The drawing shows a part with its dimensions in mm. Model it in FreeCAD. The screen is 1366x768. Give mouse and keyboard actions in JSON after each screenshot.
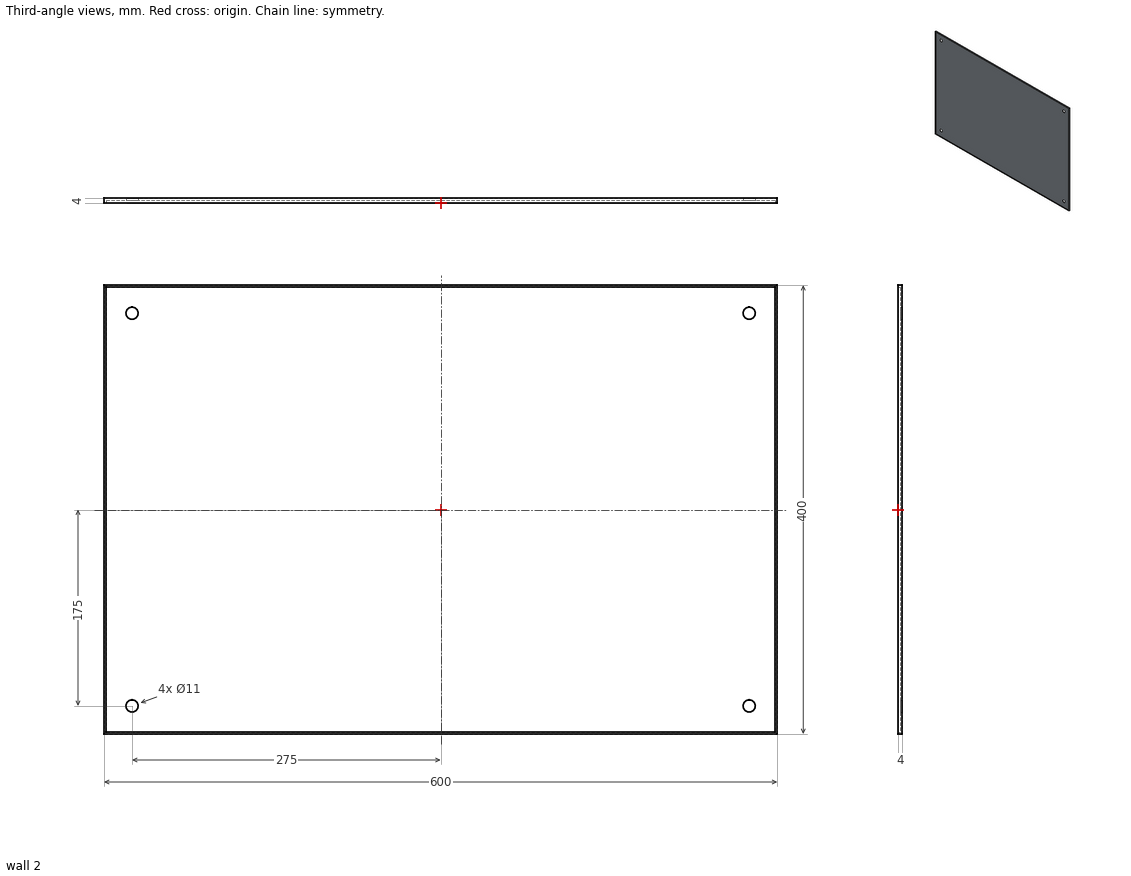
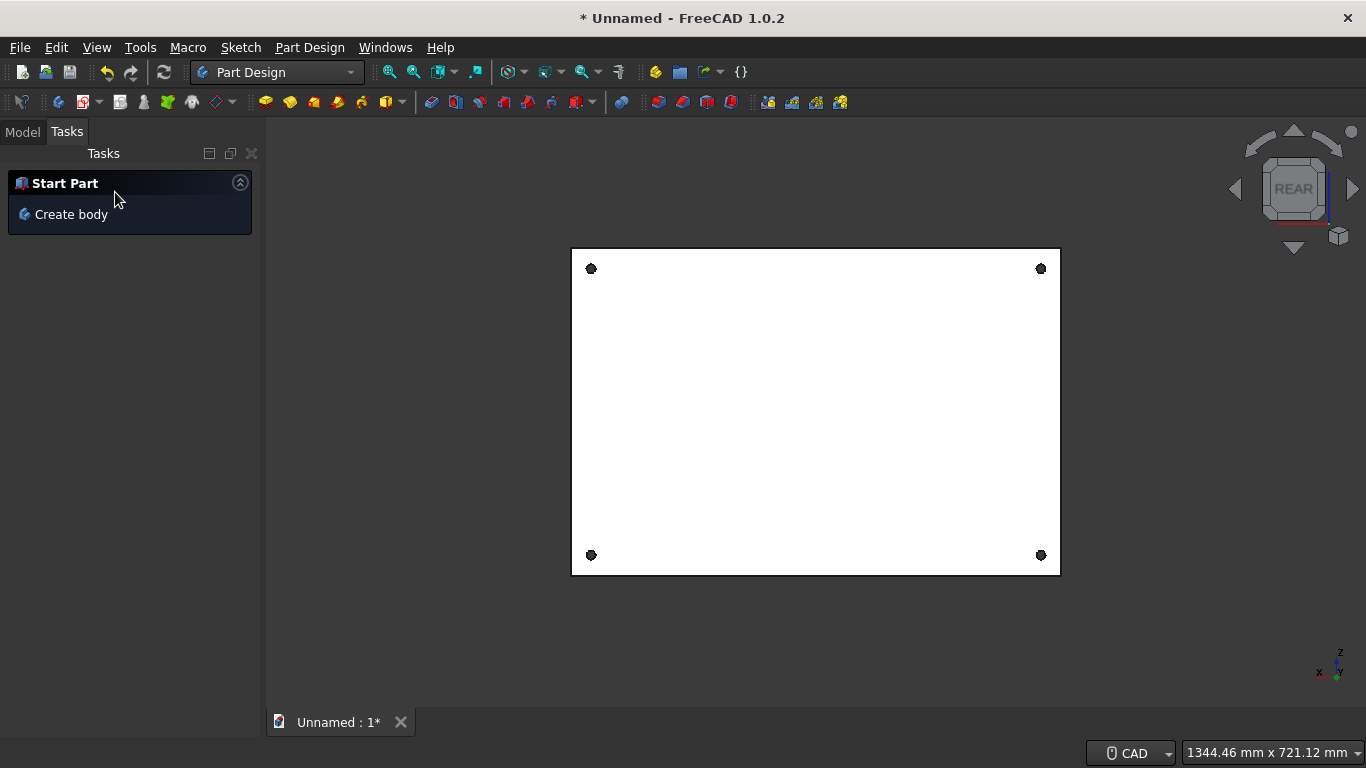
{"action": "key", "text": "0"}